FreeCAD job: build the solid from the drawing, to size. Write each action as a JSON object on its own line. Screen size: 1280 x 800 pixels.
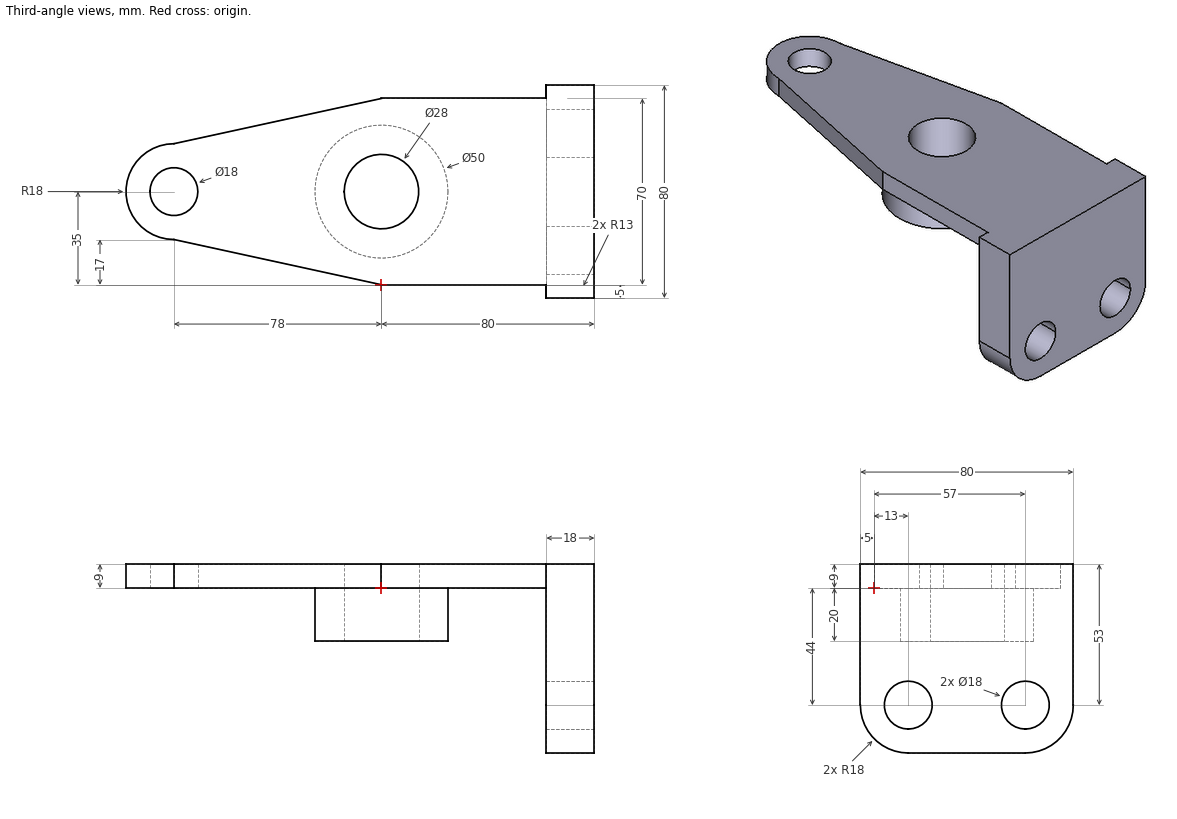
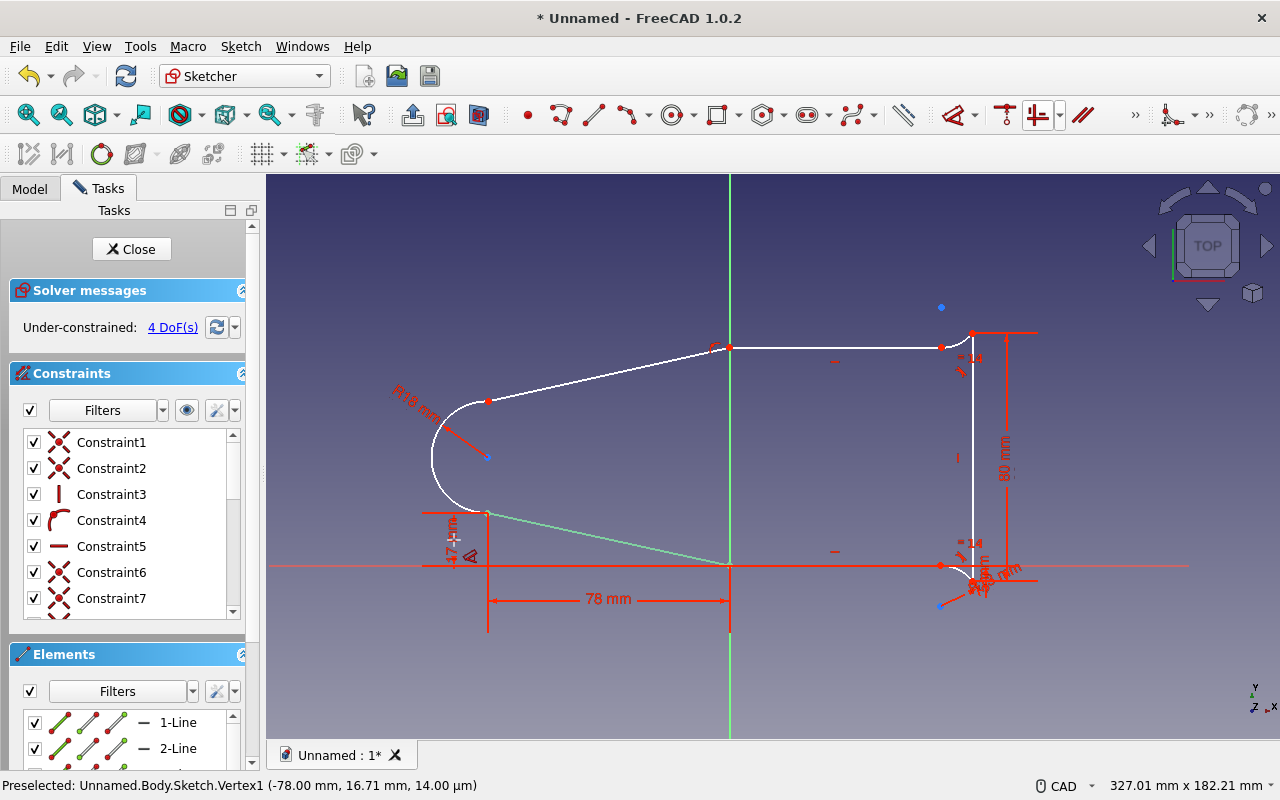
{"action": "left_click", "coordinate": [973, 581]}
{"action": "left_click", "coordinate": [851, 615]}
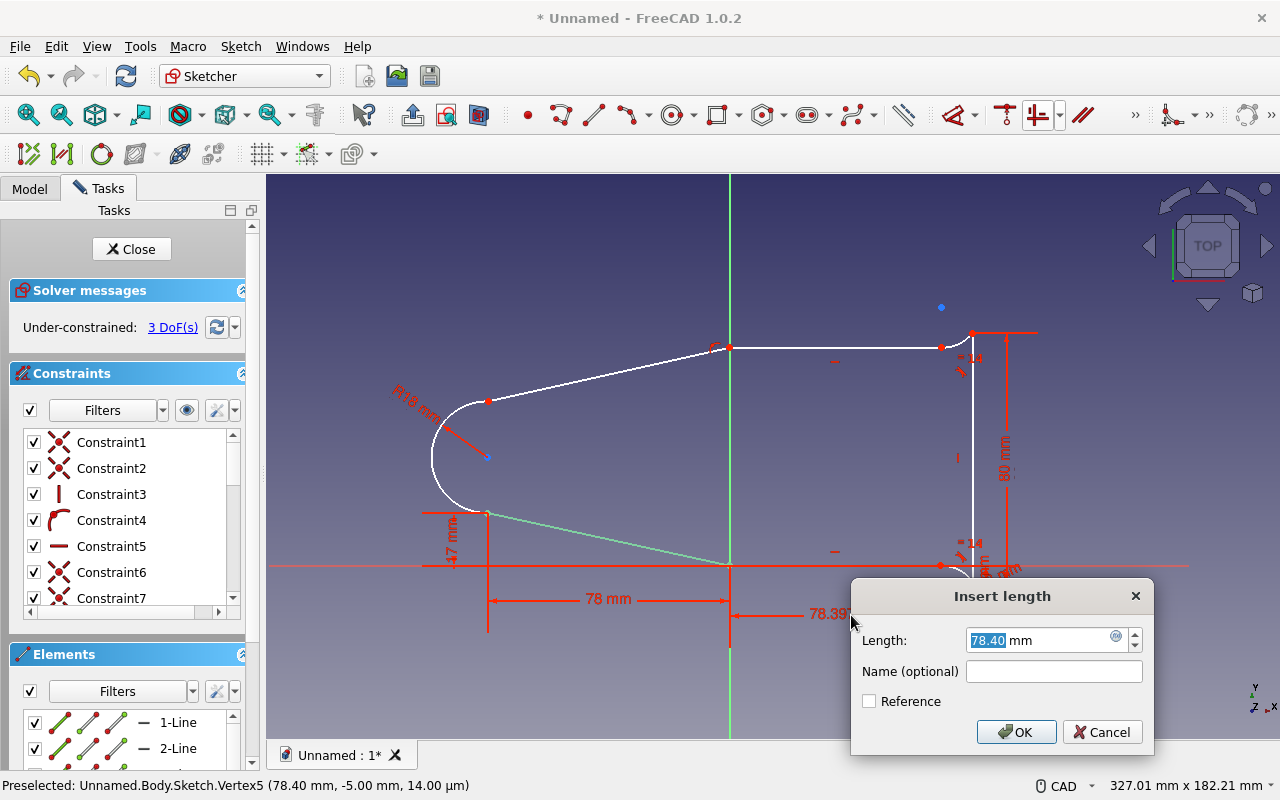
{"action": "type", "text": "80"}
{"action": "key", "text": "Return"}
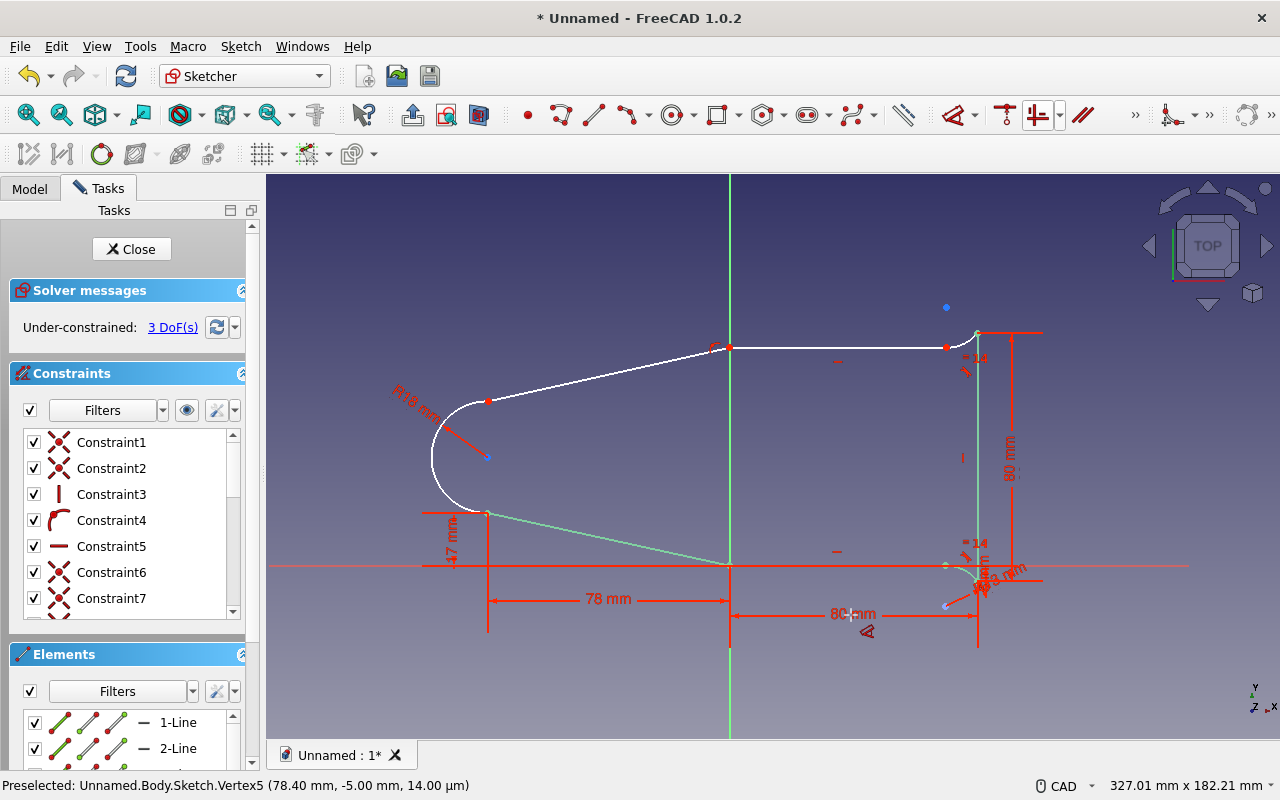
{"action": "left_click", "coordinate": [947, 348]}
{"action": "left_click", "coordinate": [696, 457]}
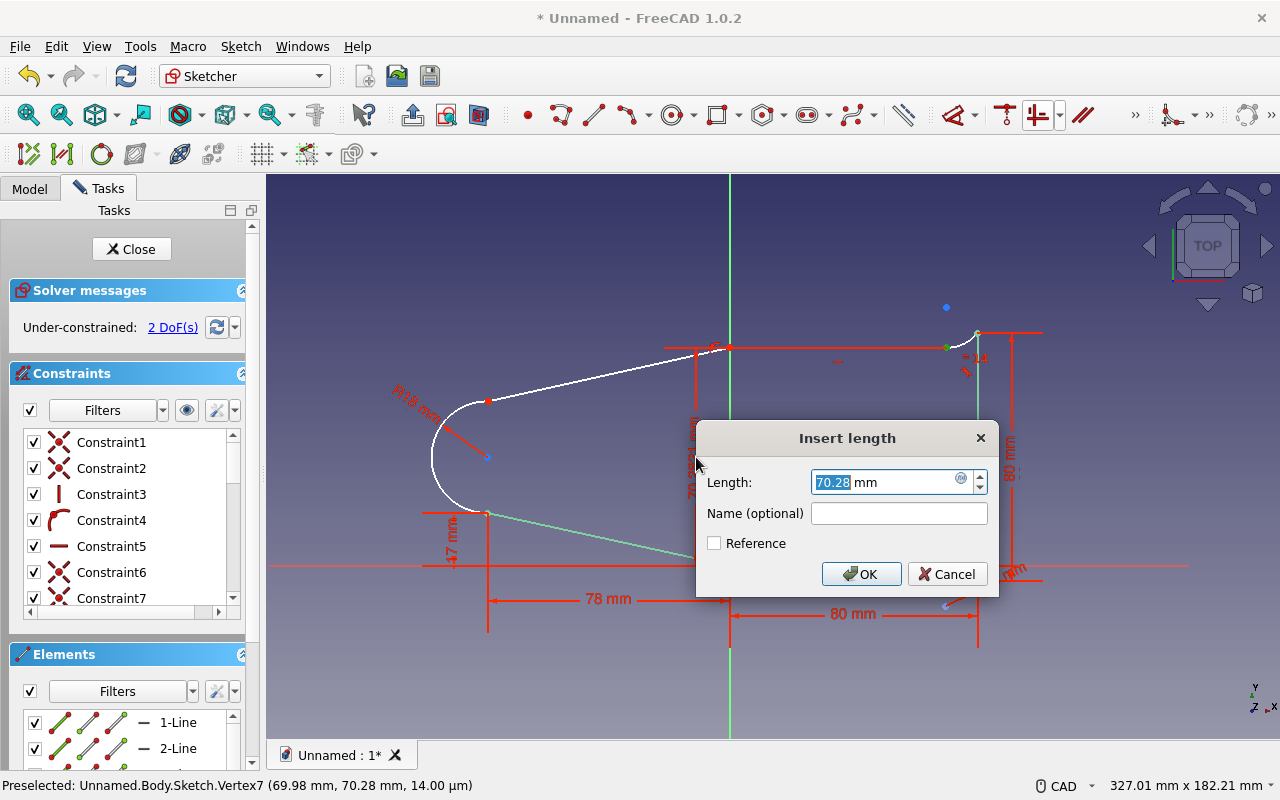
{"action": "type", "text": "70"}
{"action": "key", "text": "Return"}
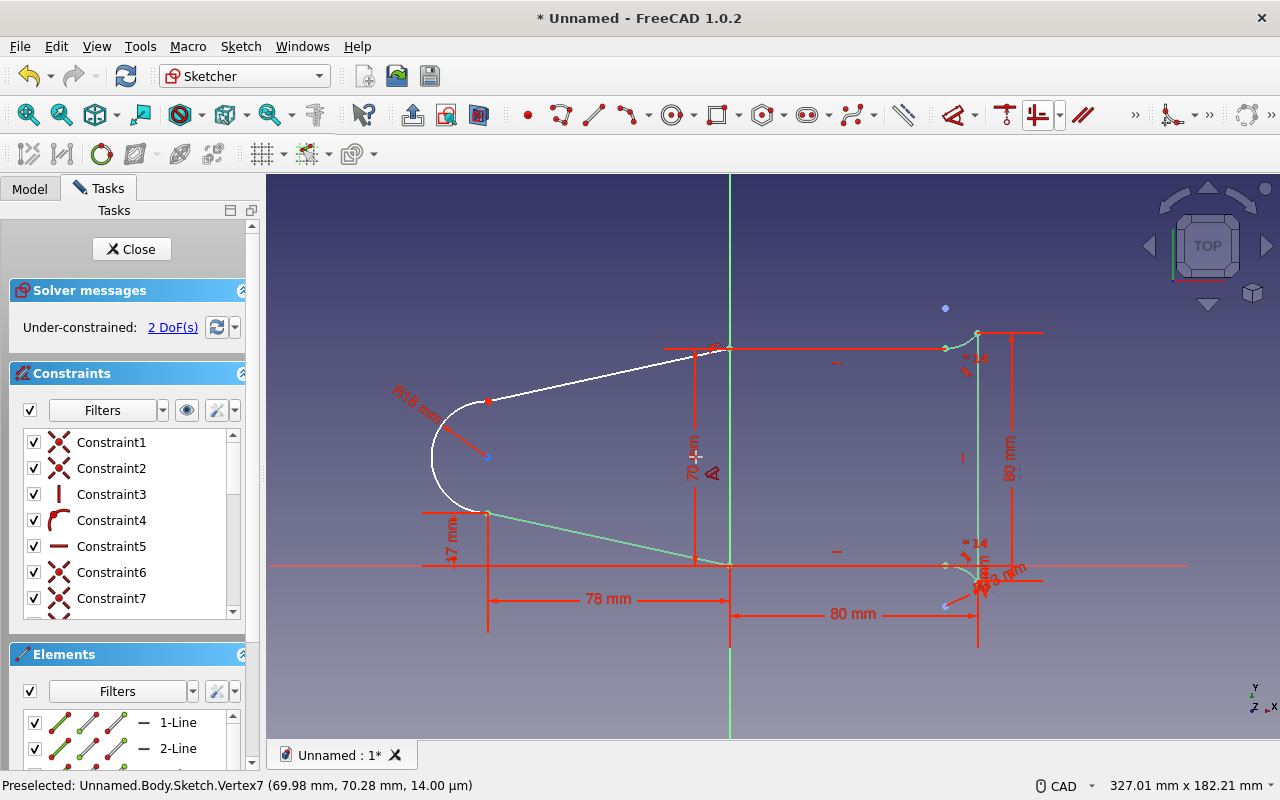
{"action": "left_click", "coordinate": [488, 401]}
{"action": "left_click", "coordinate": [524, 600]}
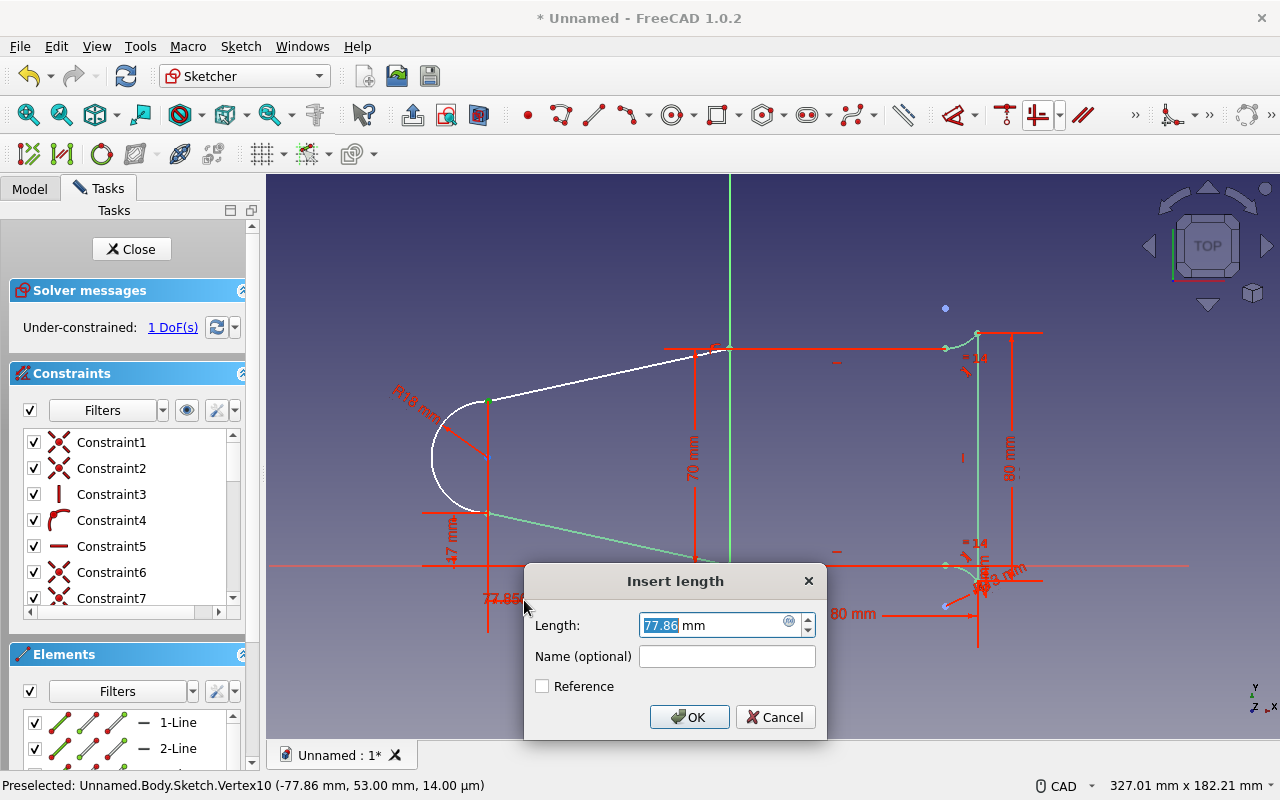
{"action": "type", "text": "78"}
{"action": "key", "text": "Return"}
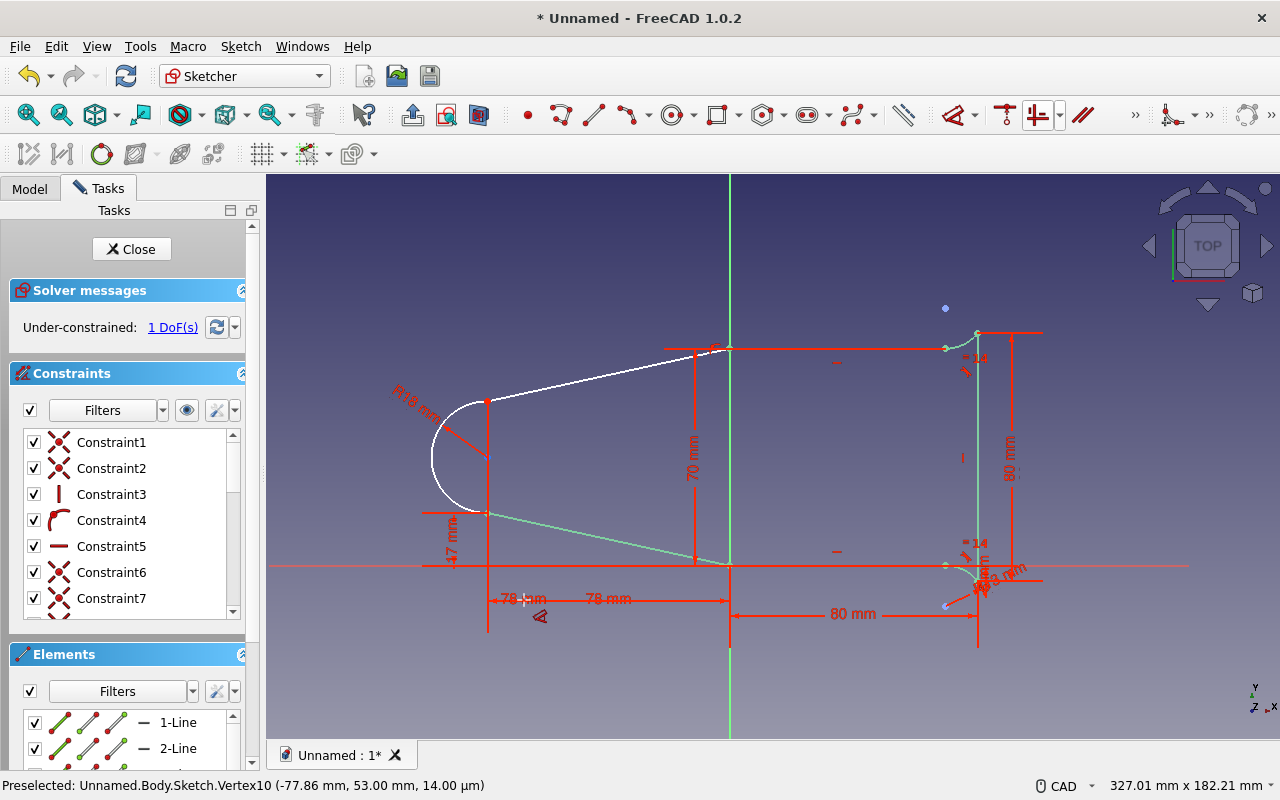
{"action": "left_click", "coordinate": [487, 457]}
{"action": "left_click", "coordinate": [693, 600]}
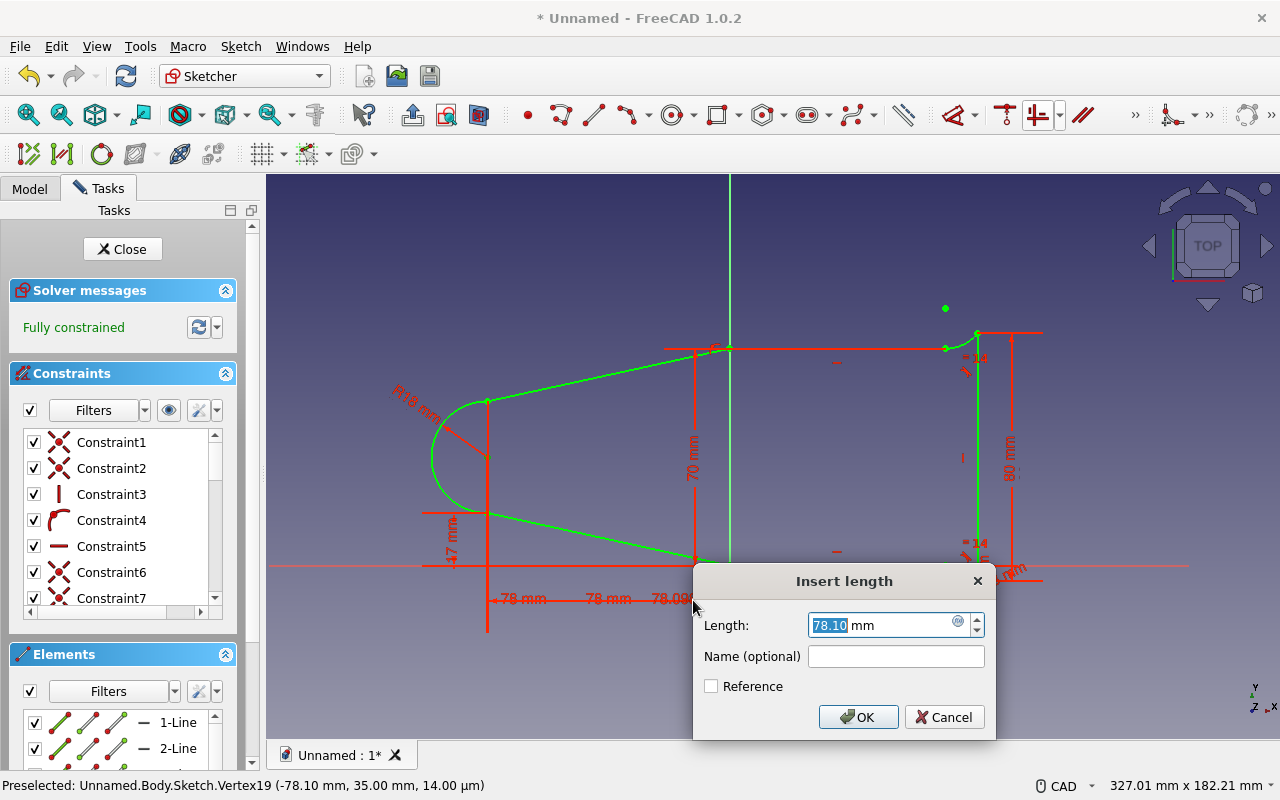
{"action": "type", "text": "78"}
{"action": "key", "text": "Return"}
{"action": "key", "text": "Escape"}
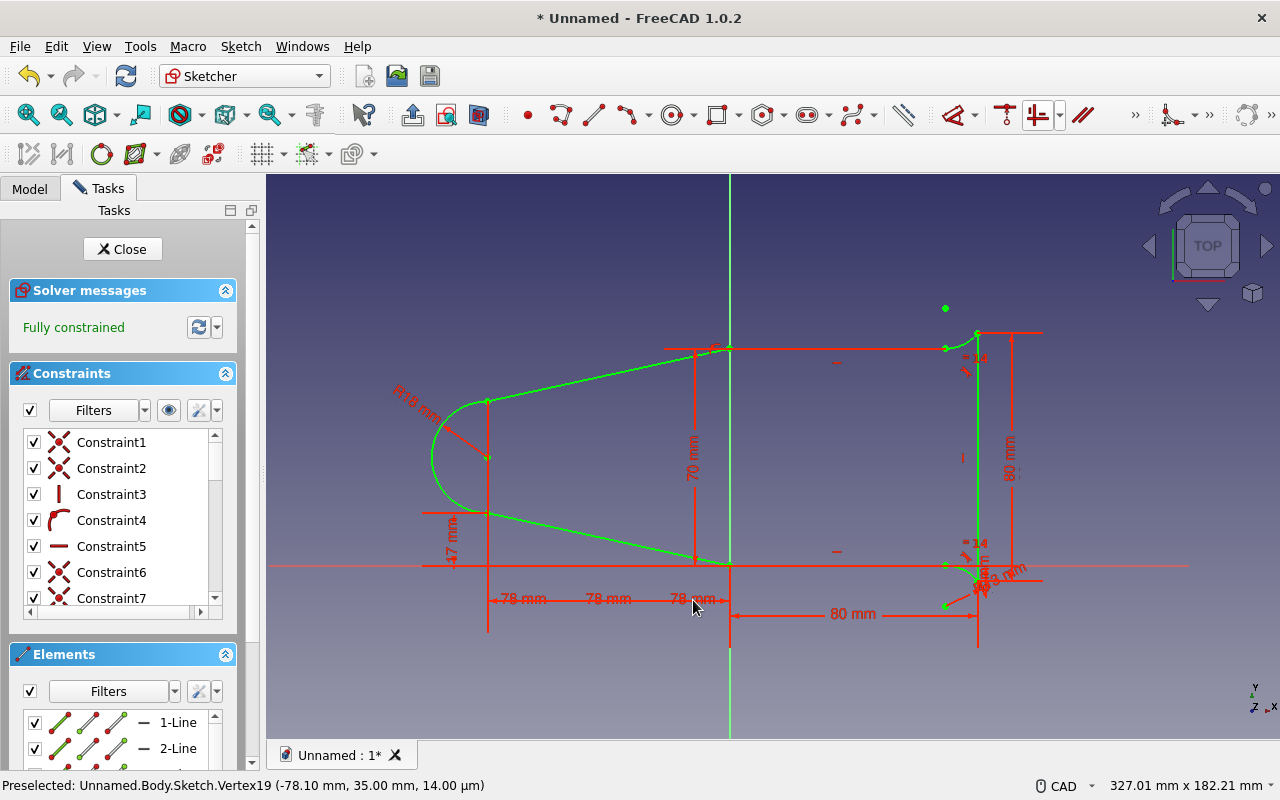
{"action": "left_click", "coordinate": [123, 249]}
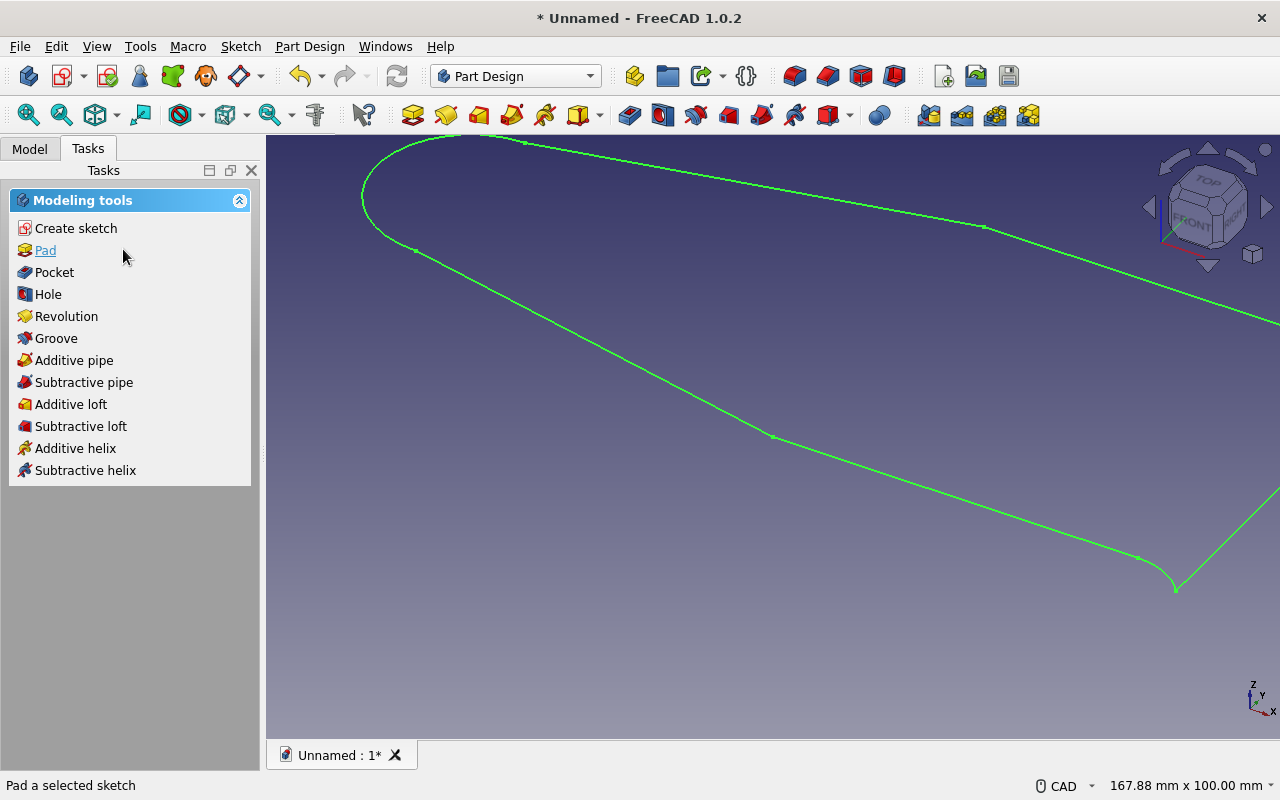
{"action": "left_click", "coordinate": [413, 116]}